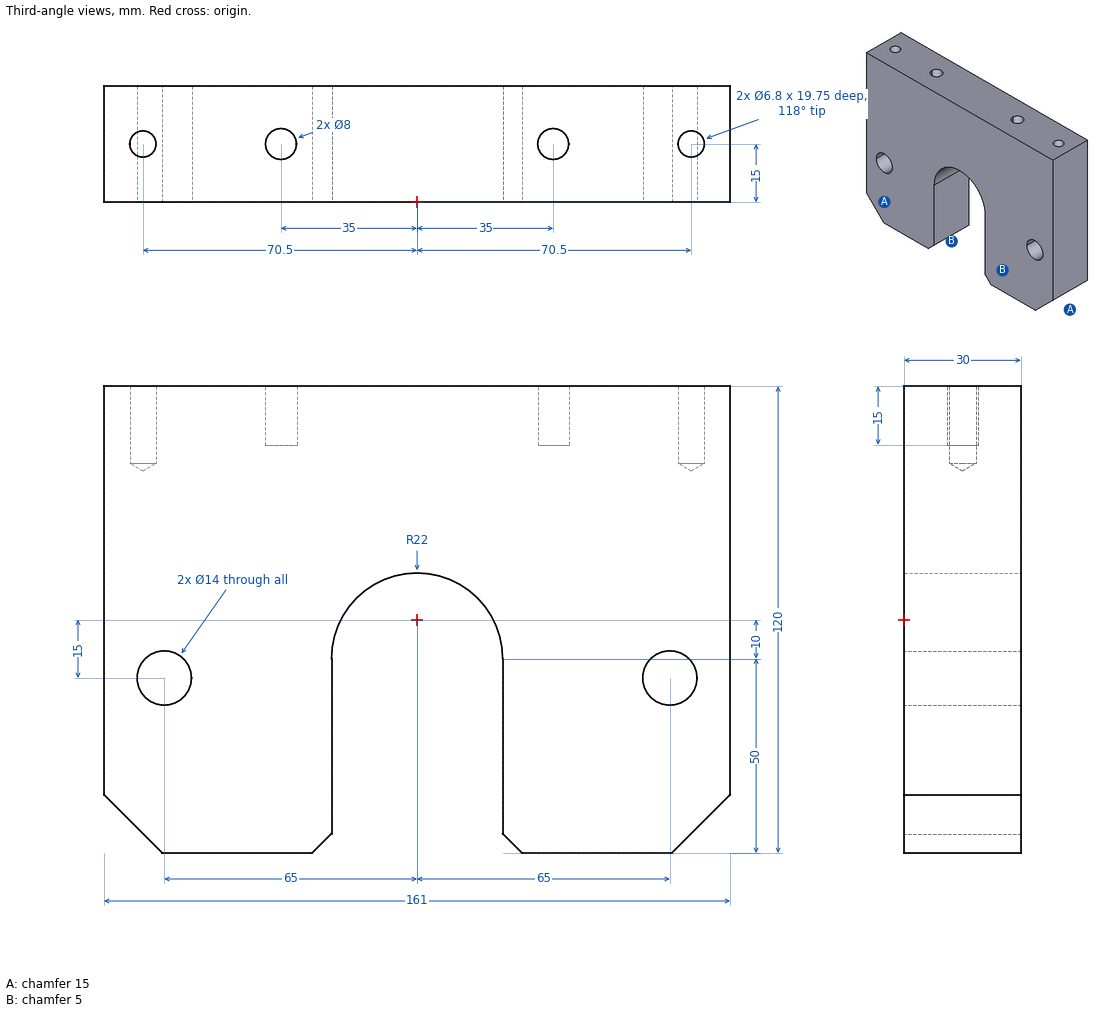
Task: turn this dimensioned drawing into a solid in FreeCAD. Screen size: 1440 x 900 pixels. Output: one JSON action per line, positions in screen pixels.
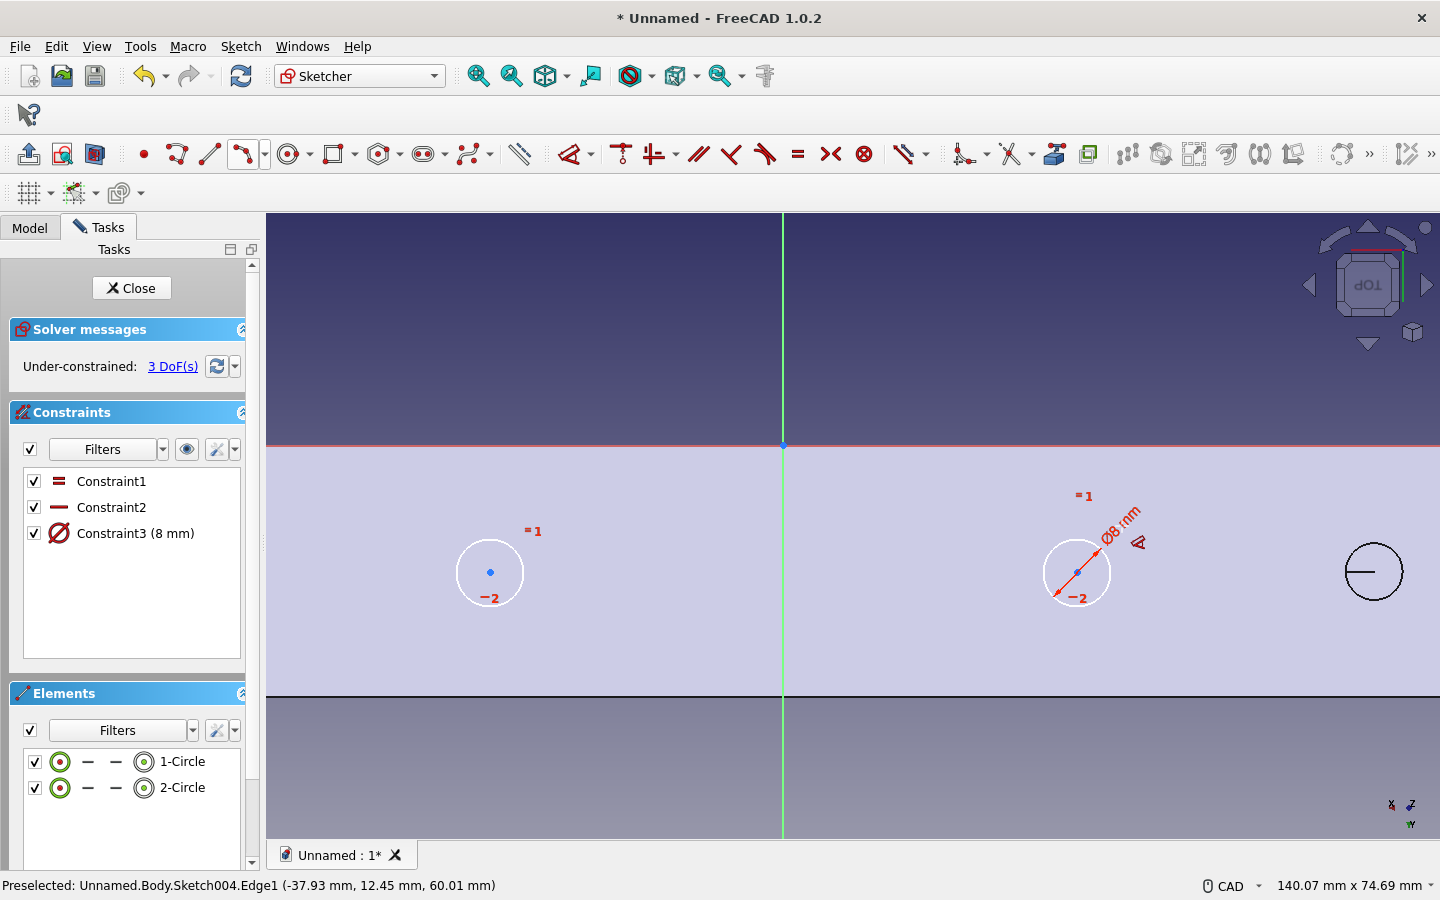
{"action": "left_click", "coordinate": [1077, 573]}
{"action": "left_click", "coordinate": [930, 412]}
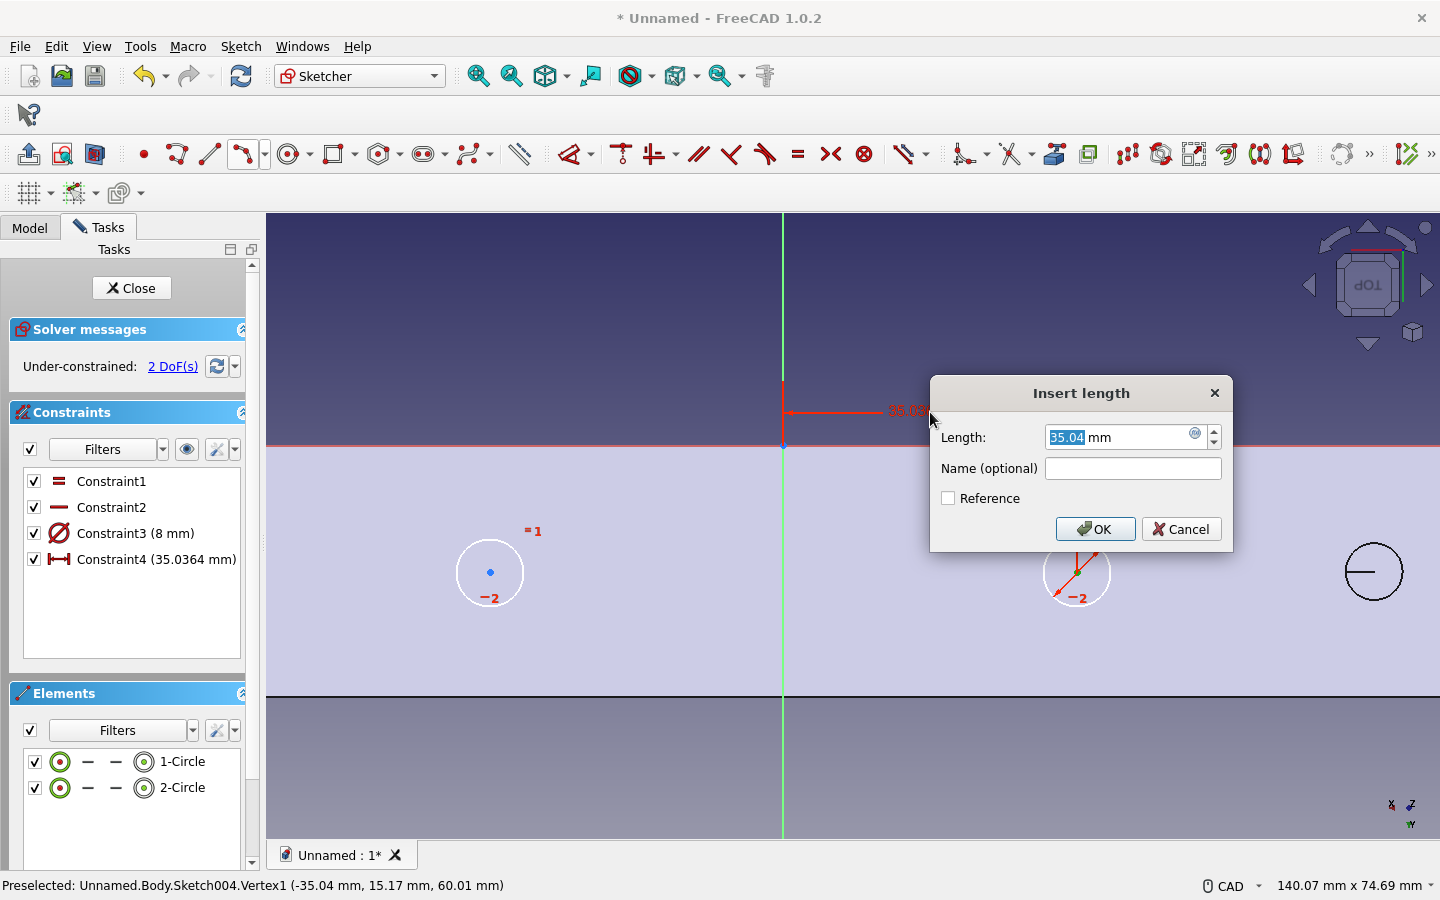
{"action": "type", "text": "35"}
{"action": "key", "text": "Return"}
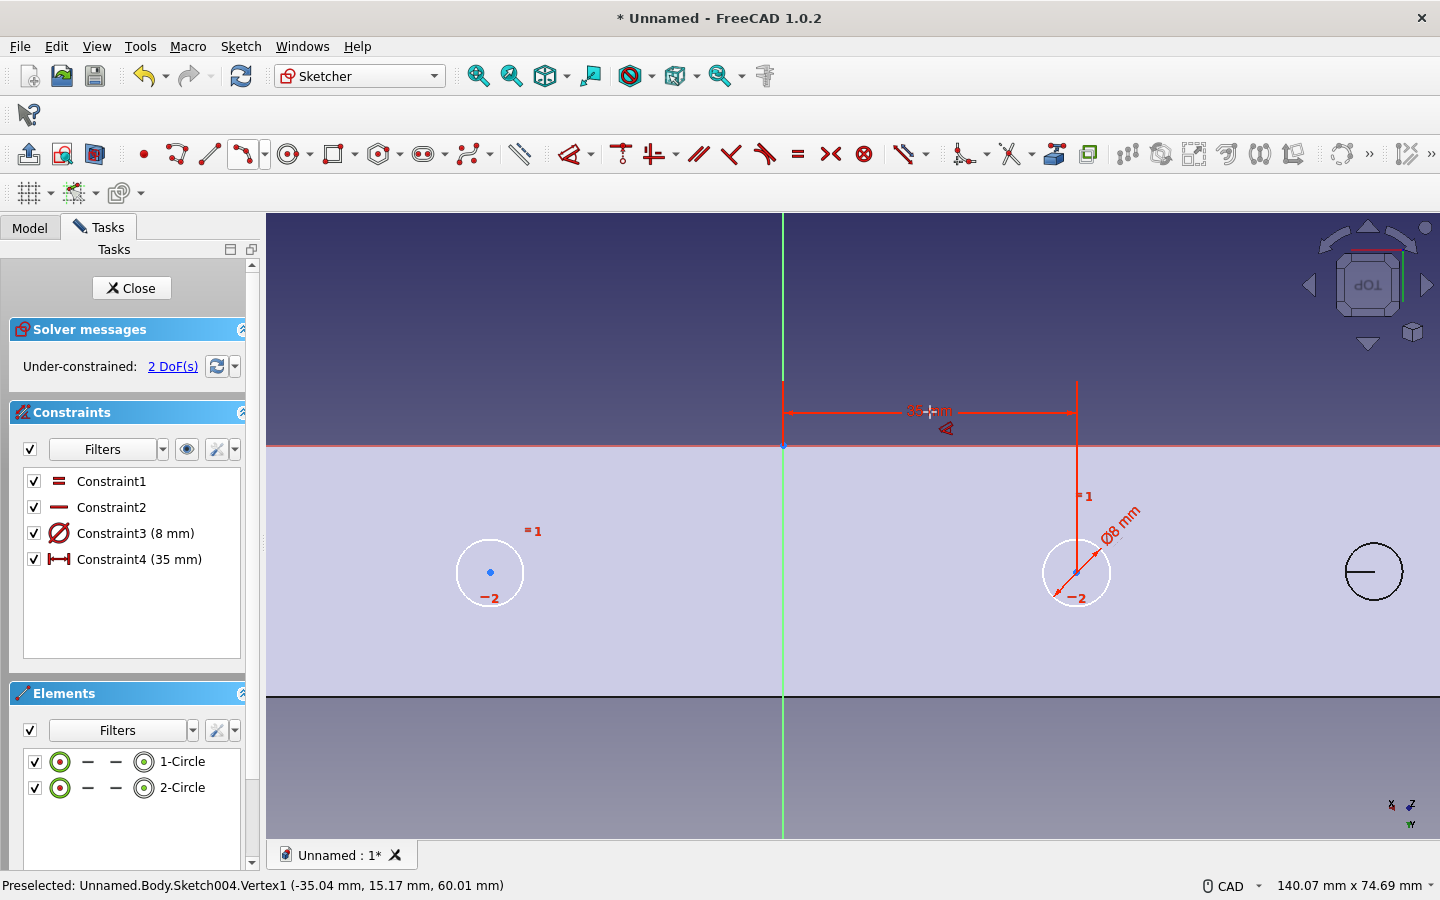
{"action": "left_click", "coordinate": [1077, 573]}
{"action": "left_click", "coordinate": [1111, 480]}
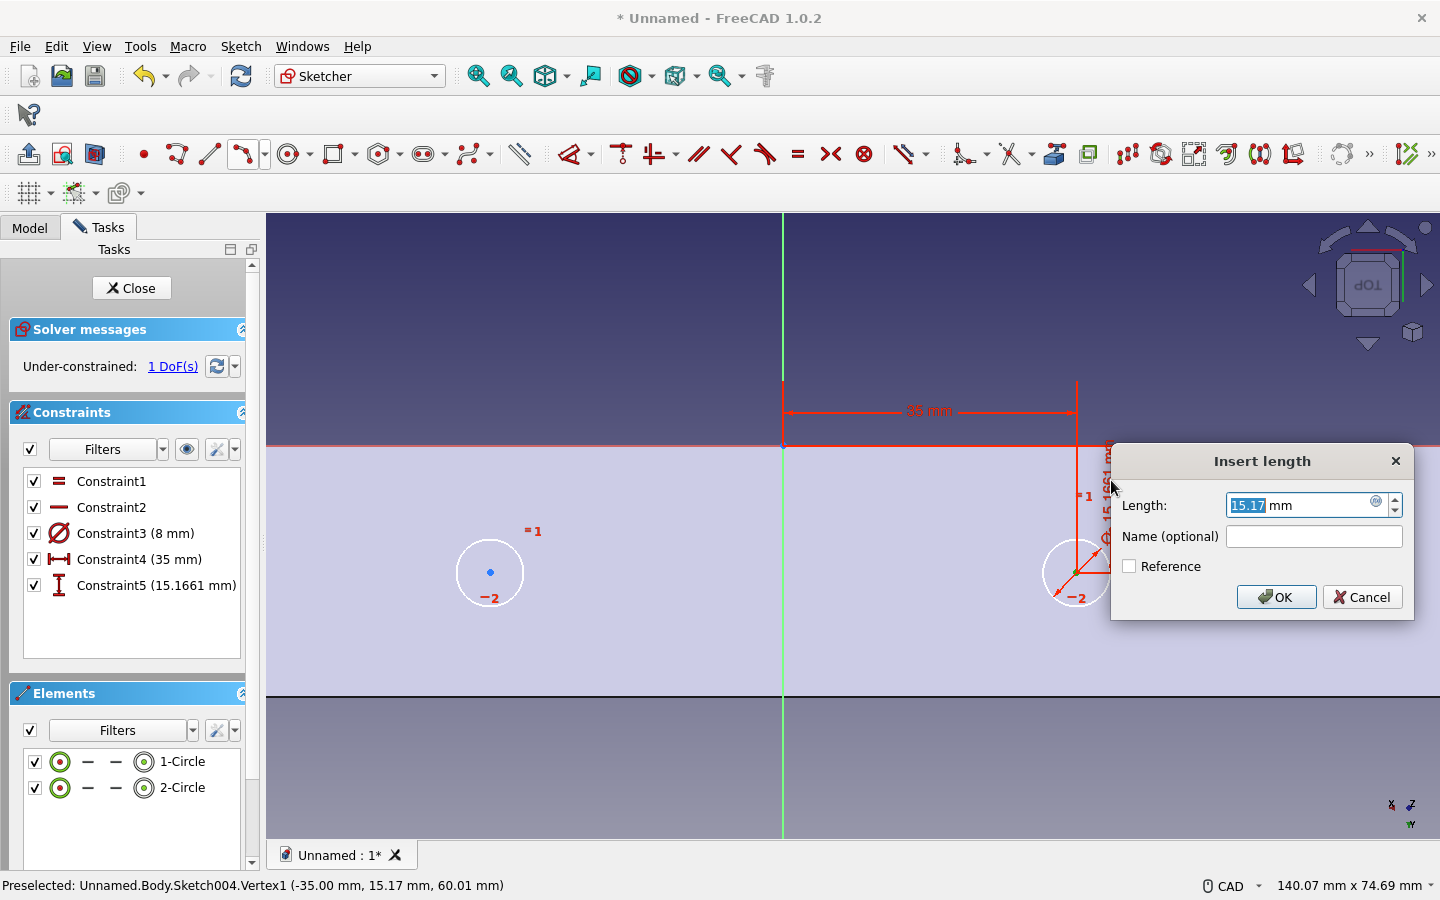
{"action": "type", "text": "15"}
{"action": "key", "text": "Return"}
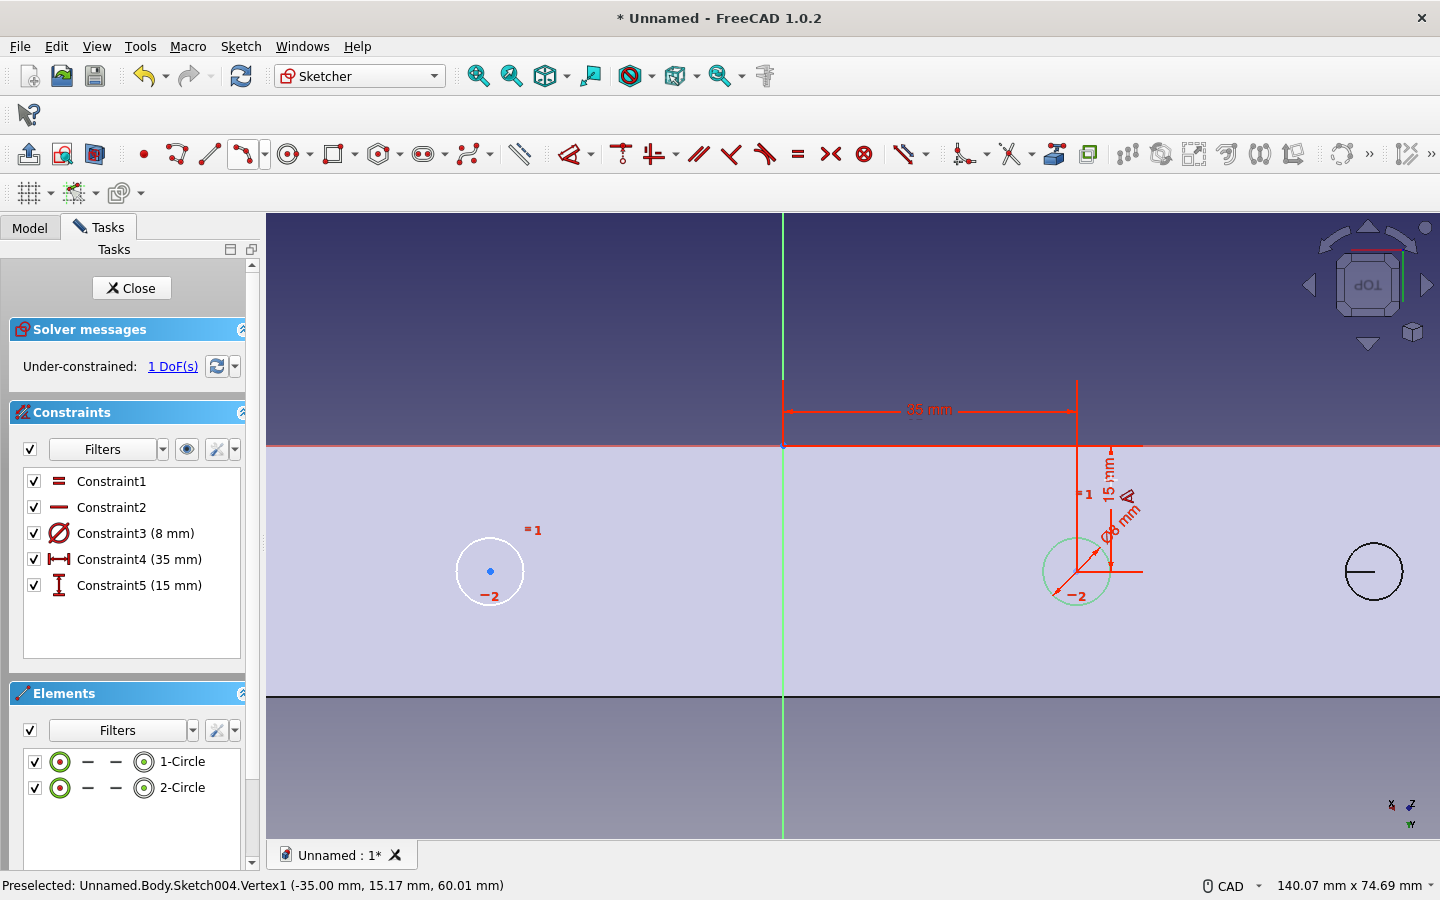
{"action": "left_click", "coordinate": [490, 572]}
{"action": "left_click", "coordinate": [637, 412]}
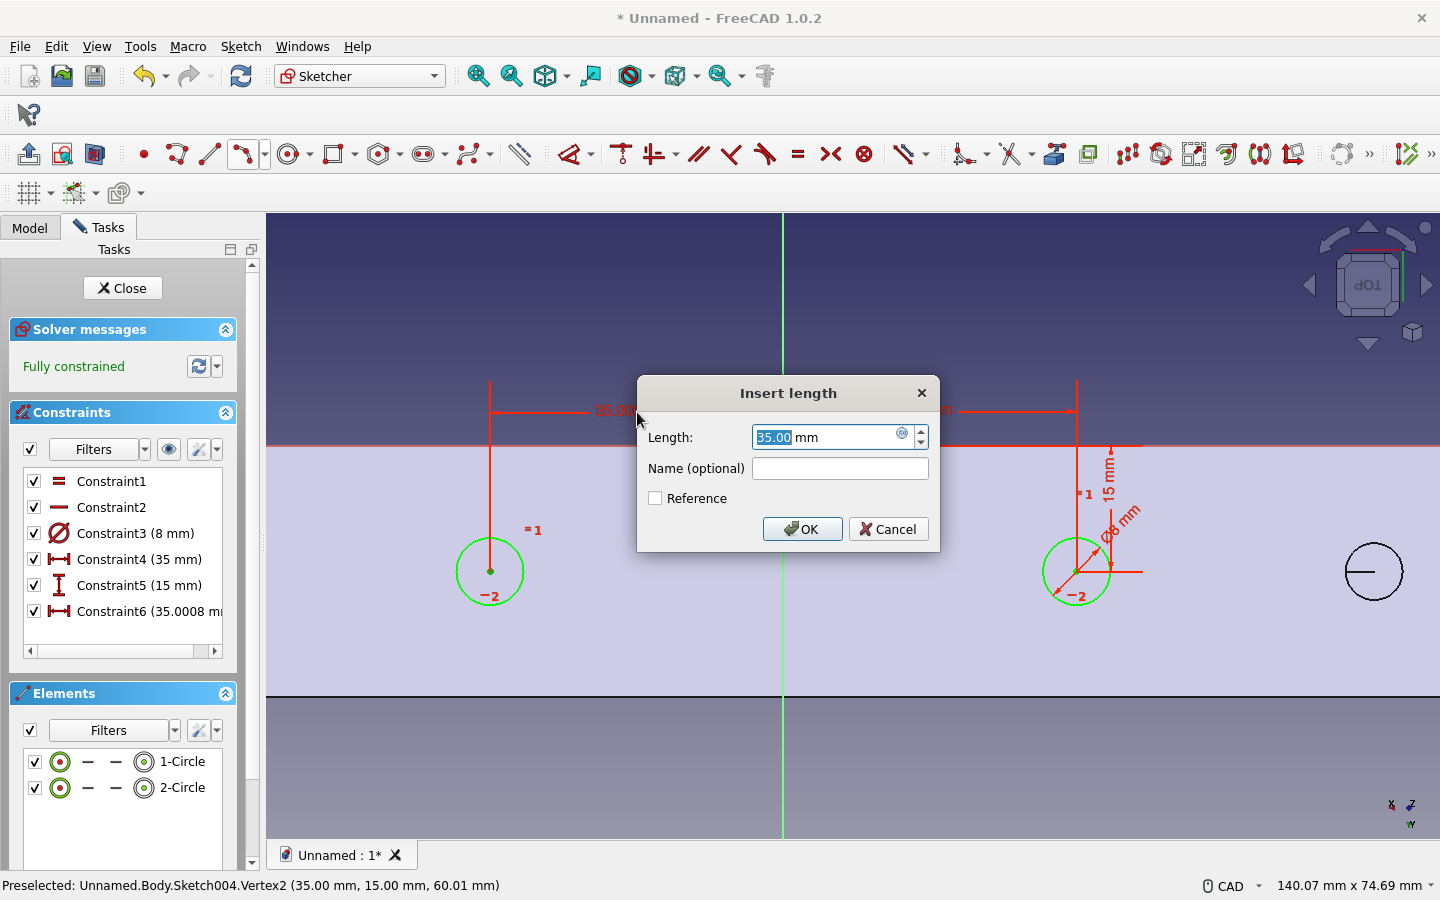
{"action": "type", "text": "35"}
{"action": "key", "text": "Return"}
{"action": "key", "text": "Escape"}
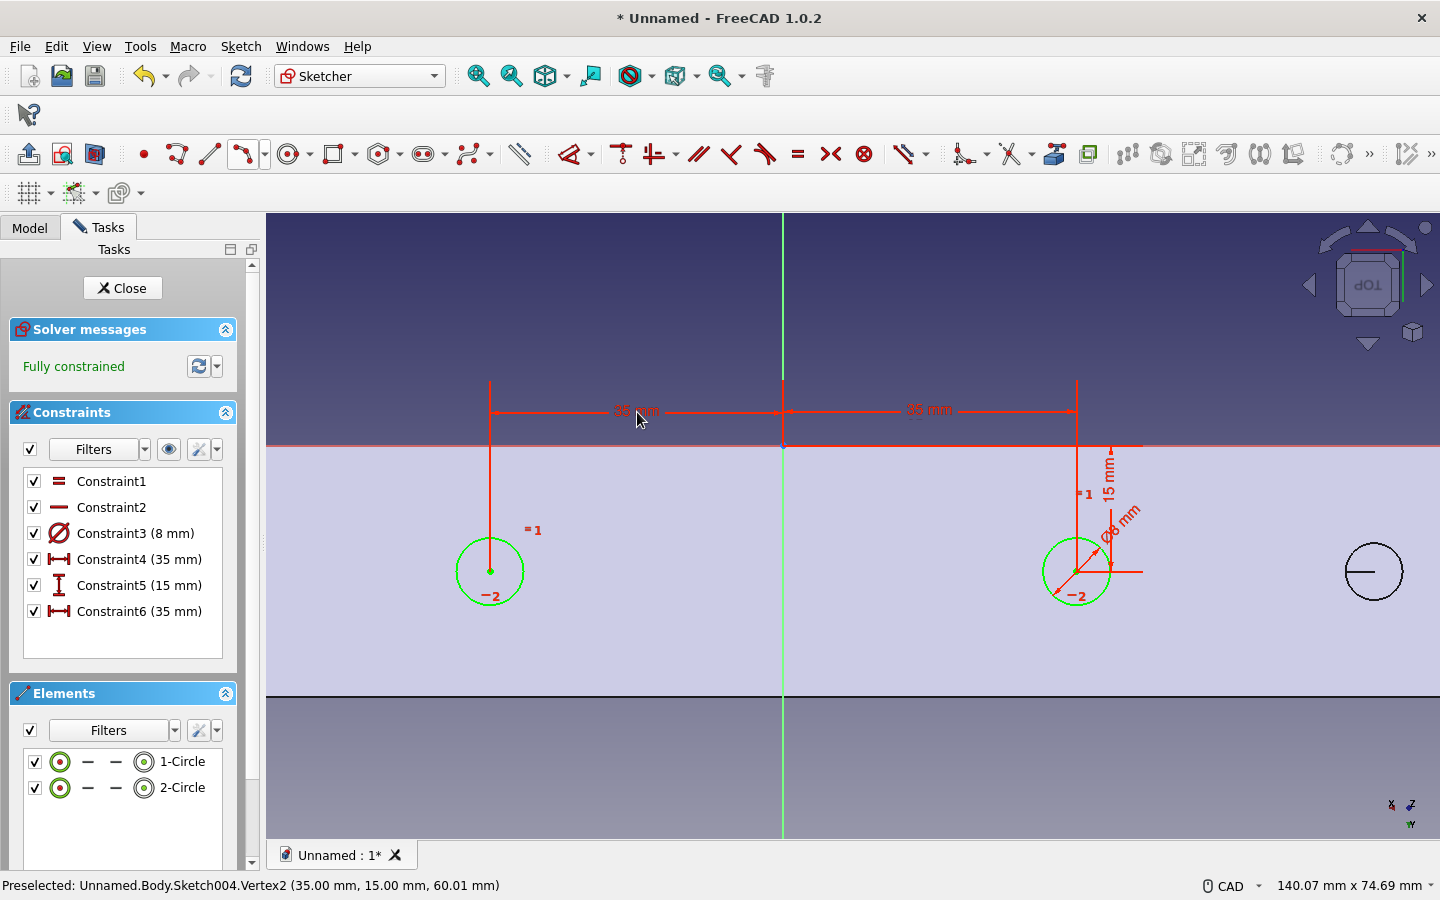
{"action": "left_click", "coordinate": [123, 288]}